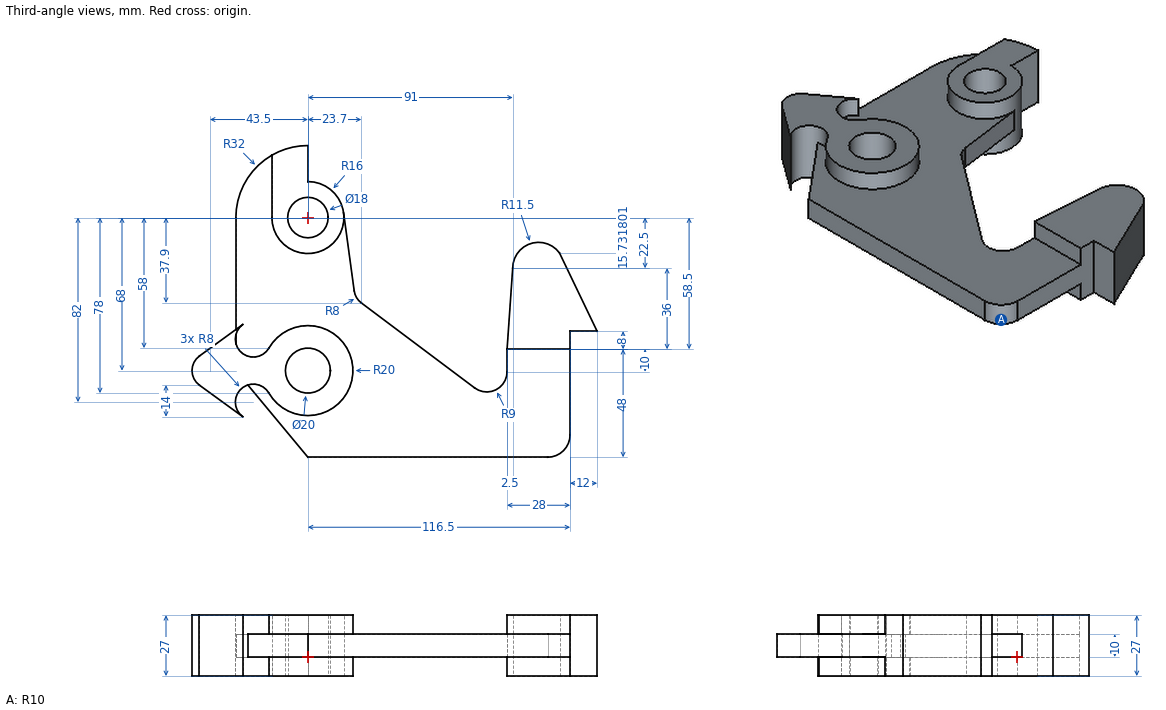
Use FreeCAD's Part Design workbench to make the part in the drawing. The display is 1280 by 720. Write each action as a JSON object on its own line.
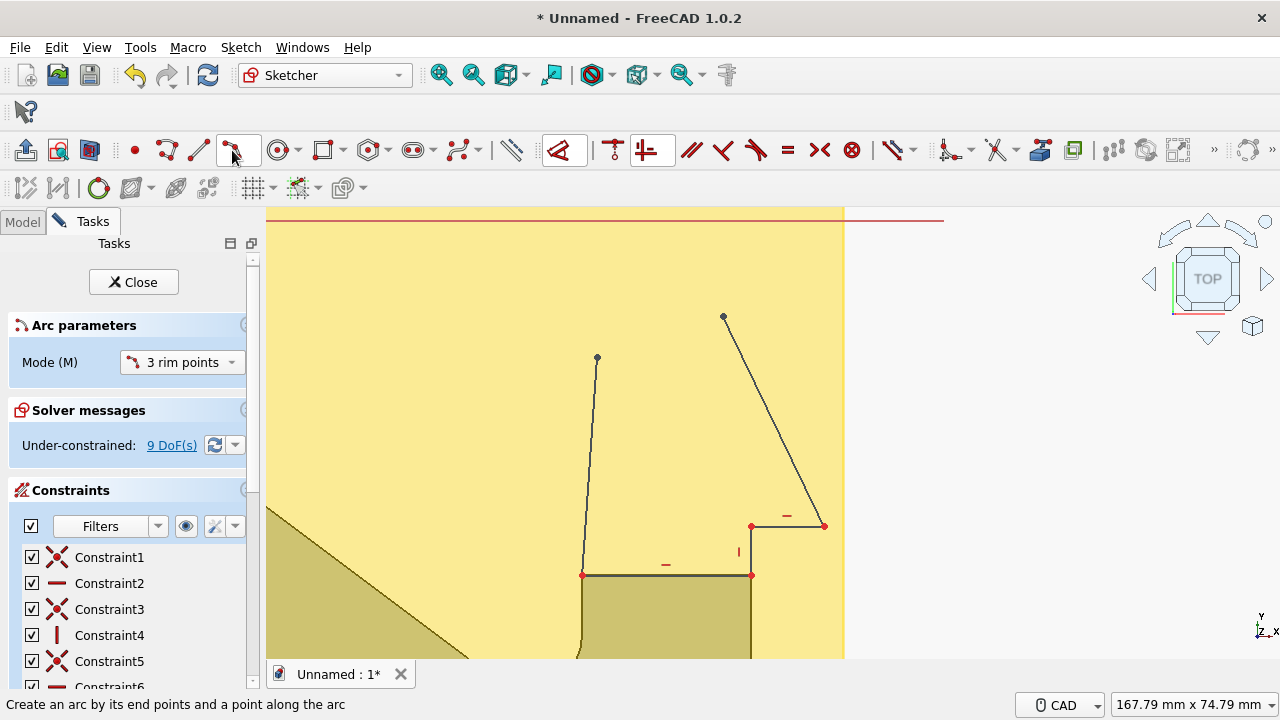
{"action": "left_click", "coordinate": [723, 317]}
{"action": "left_click", "coordinate": [597, 358]}
{"action": "left_click", "coordinate": [645, 291]}
{"action": "key", "text": "Escape"}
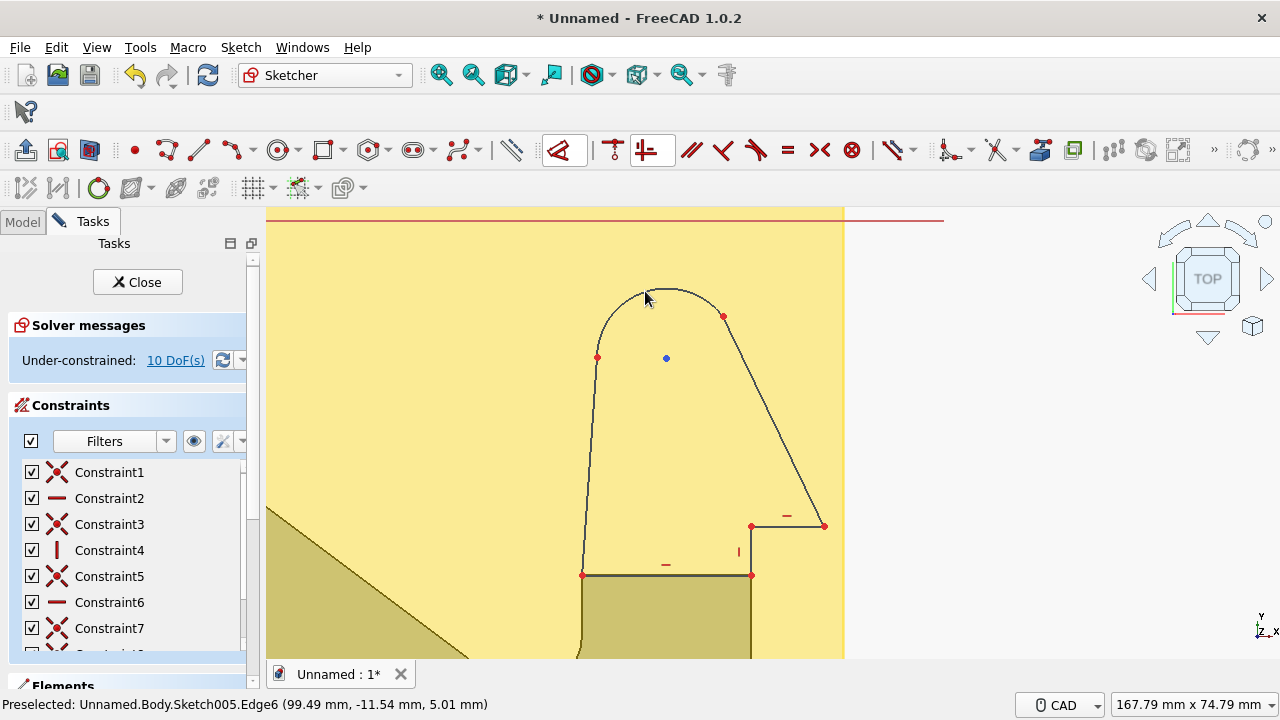
{"action": "left_click", "coordinate": [680, 290]}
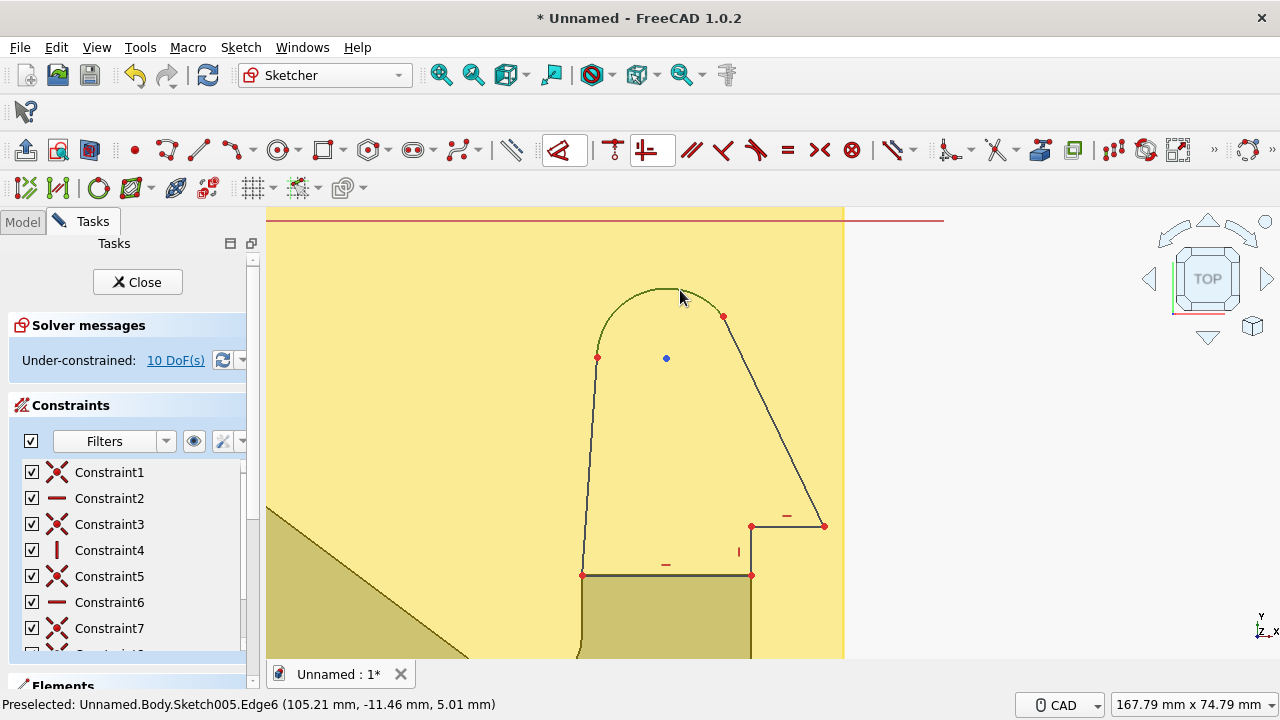
{"action": "key", "text": "k r"}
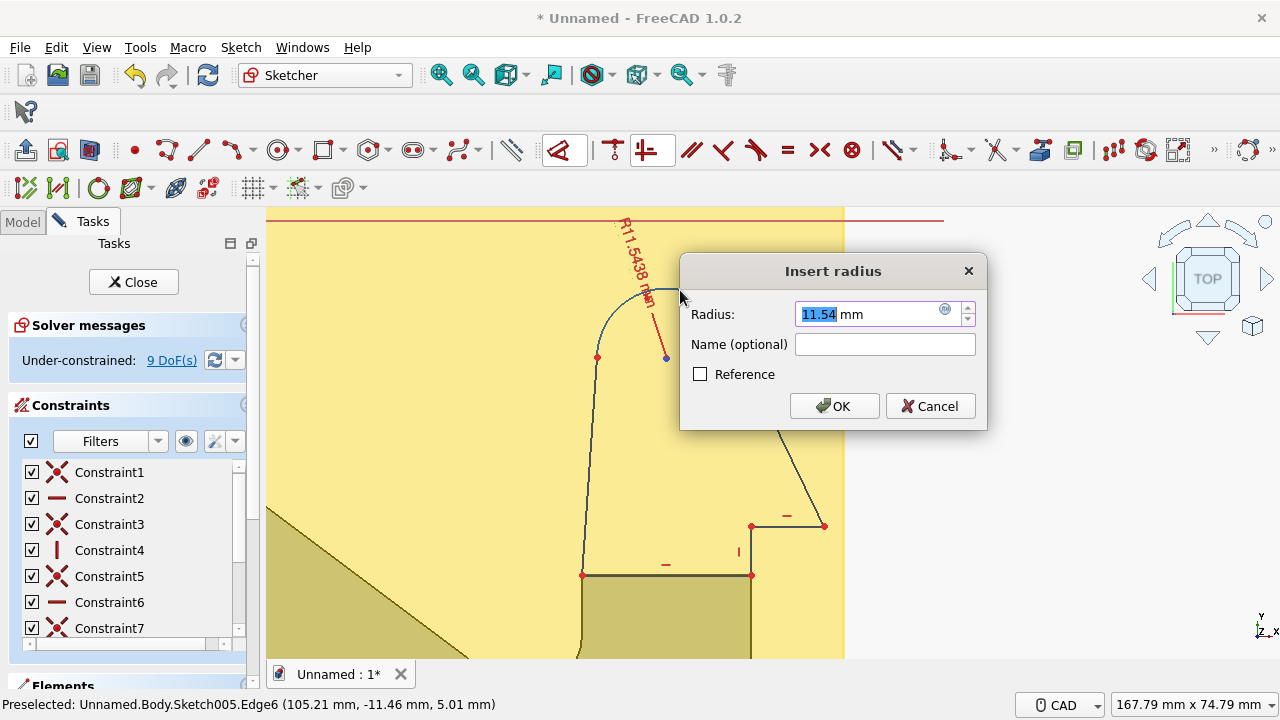
{"action": "type", "text": "11.5"}
{"action": "key", "text": "Return"}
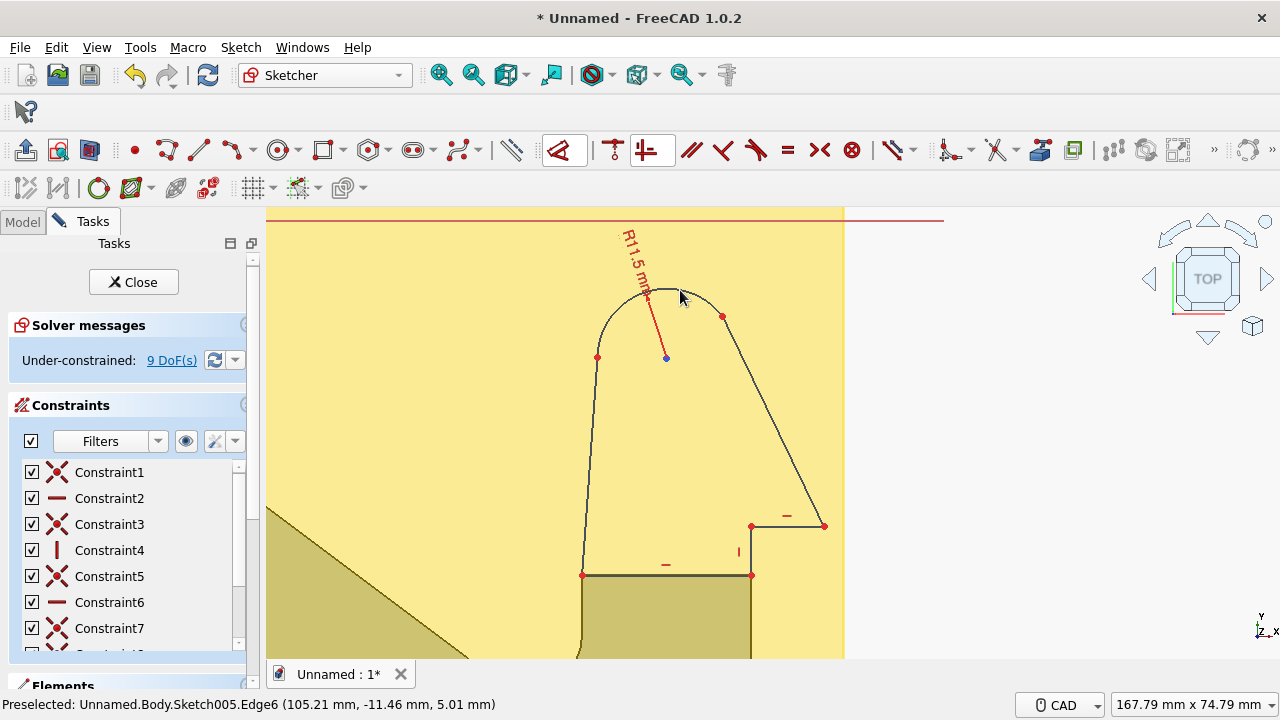
{"action": "left_click", "coordinate": [751, 561]}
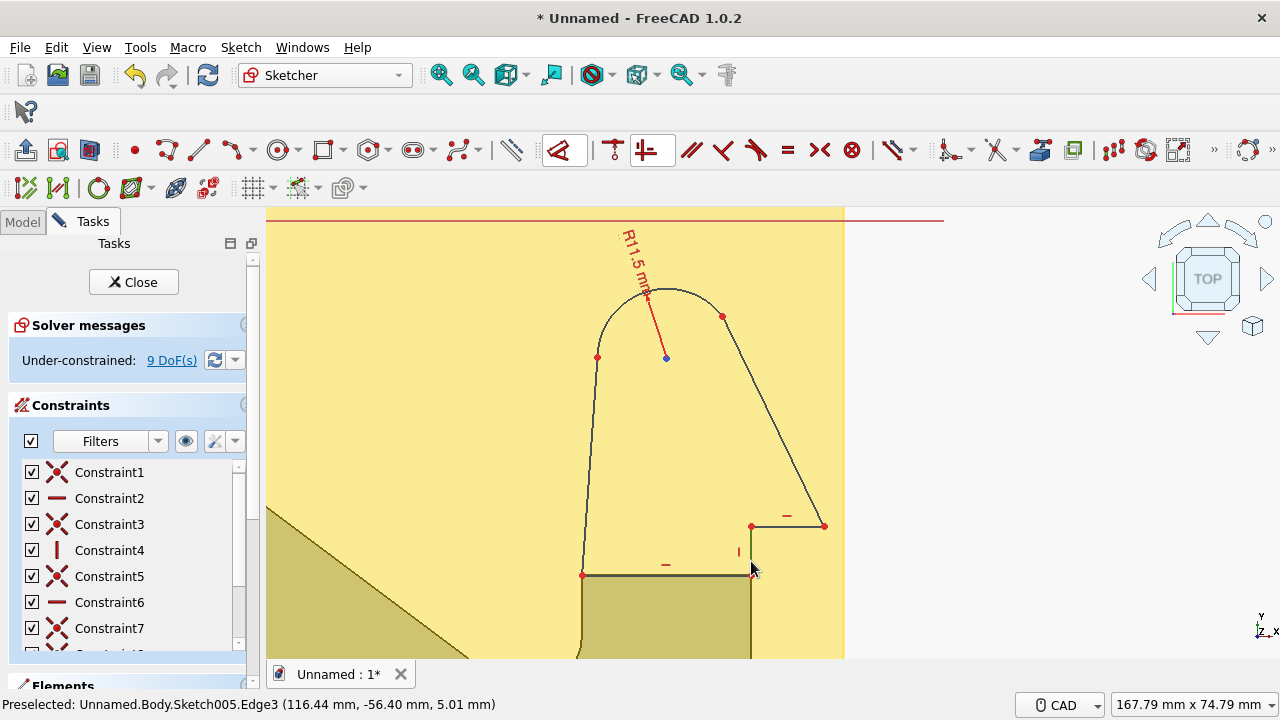
{"action": "key", "text": "i"}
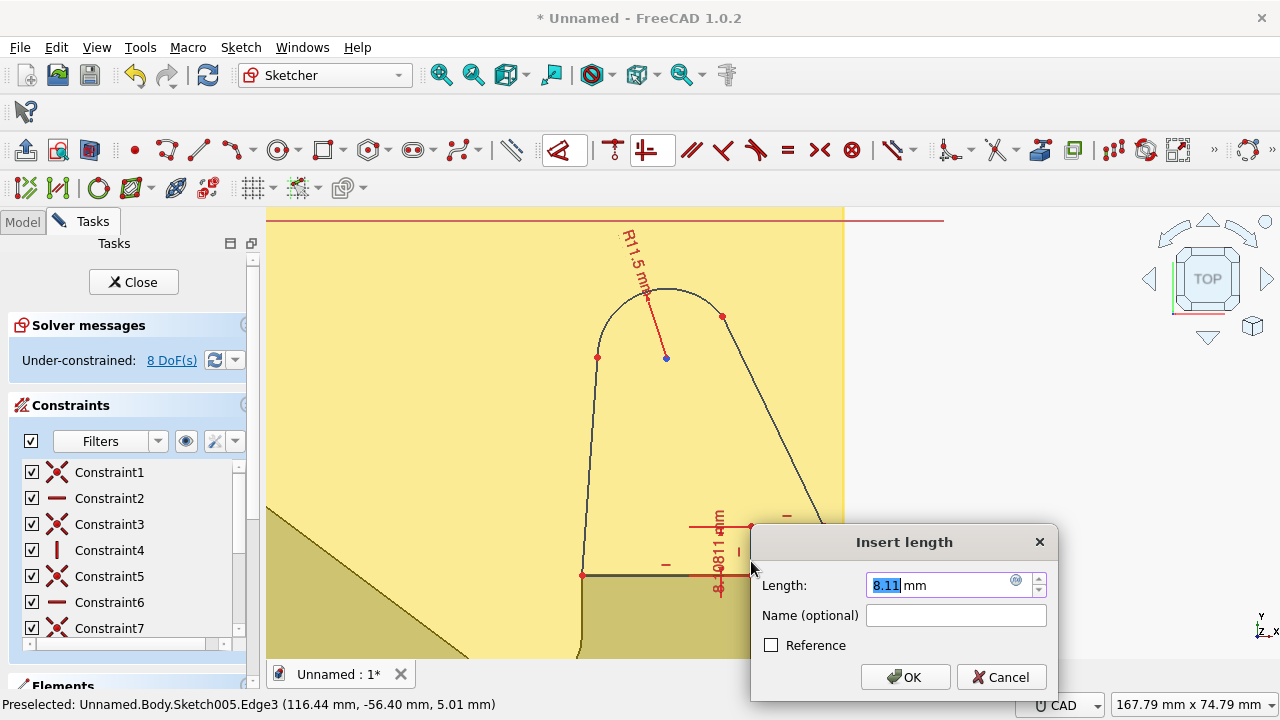
{"action": "type", "text": "8"}
{"action": "key", "text": "Return"}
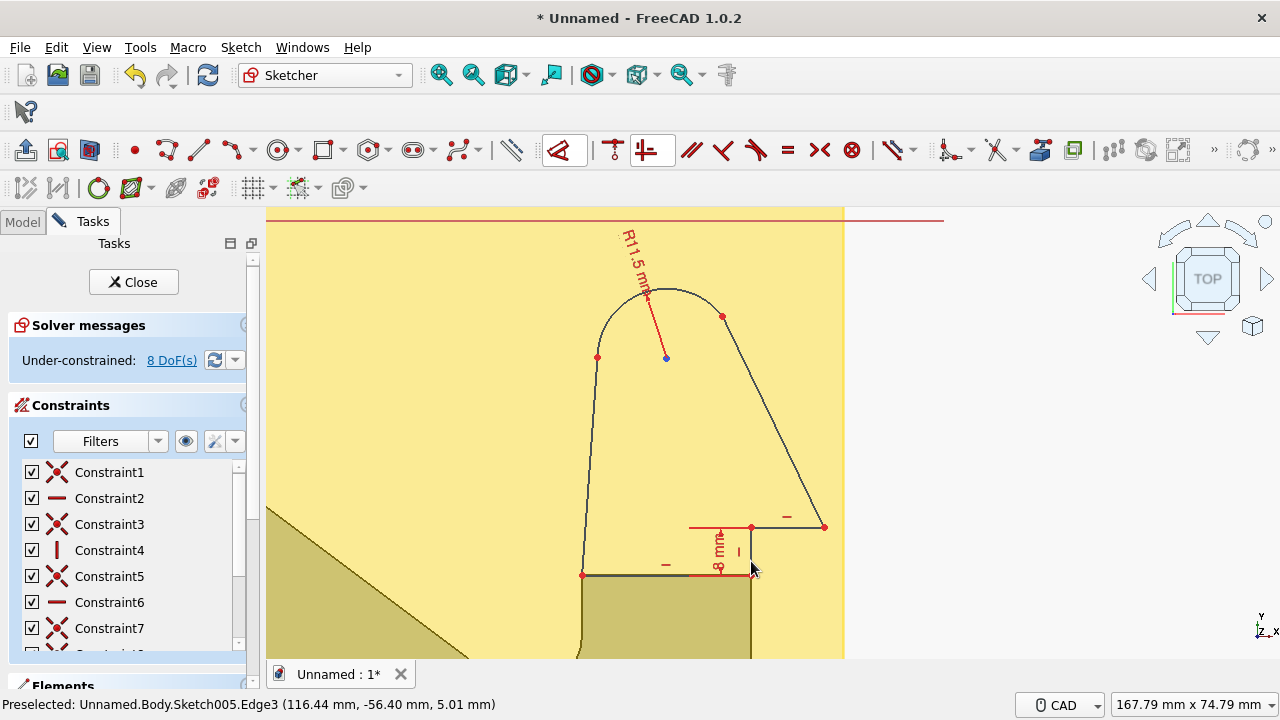
{"action": "left_click", "coordinate": [633, 576]}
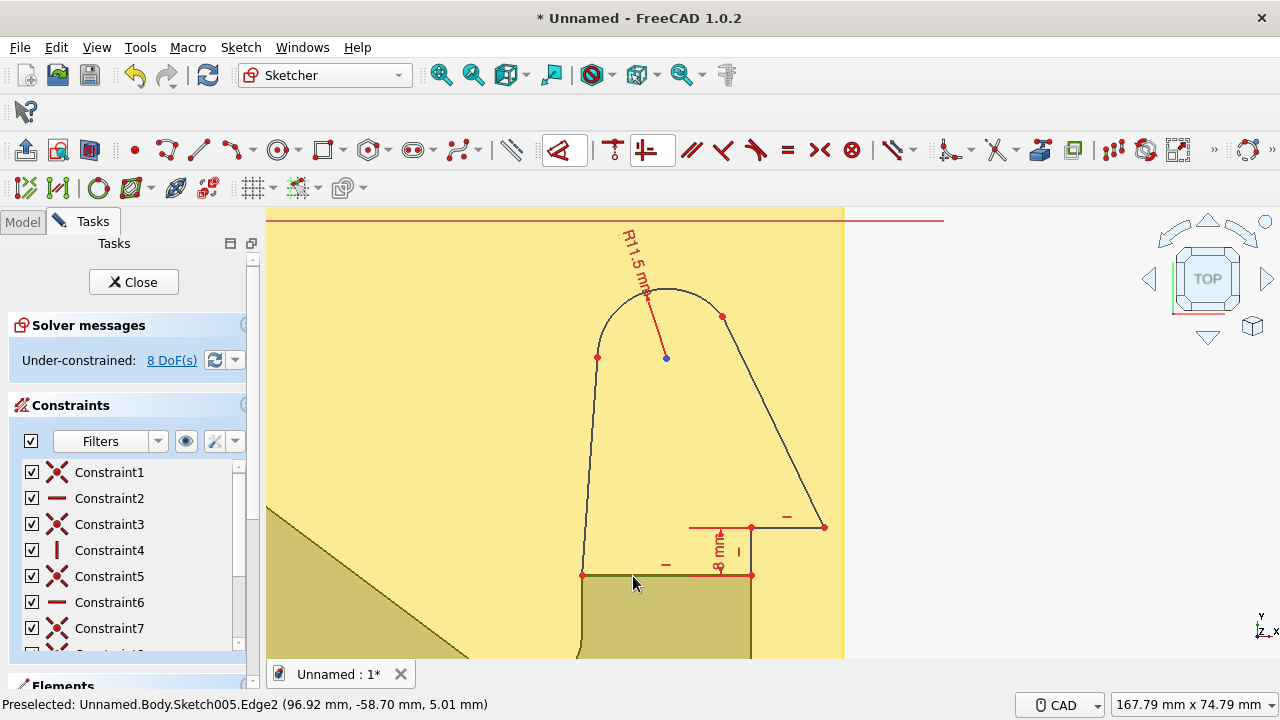
{"action": "left_click", "coordinate": [582, 150]}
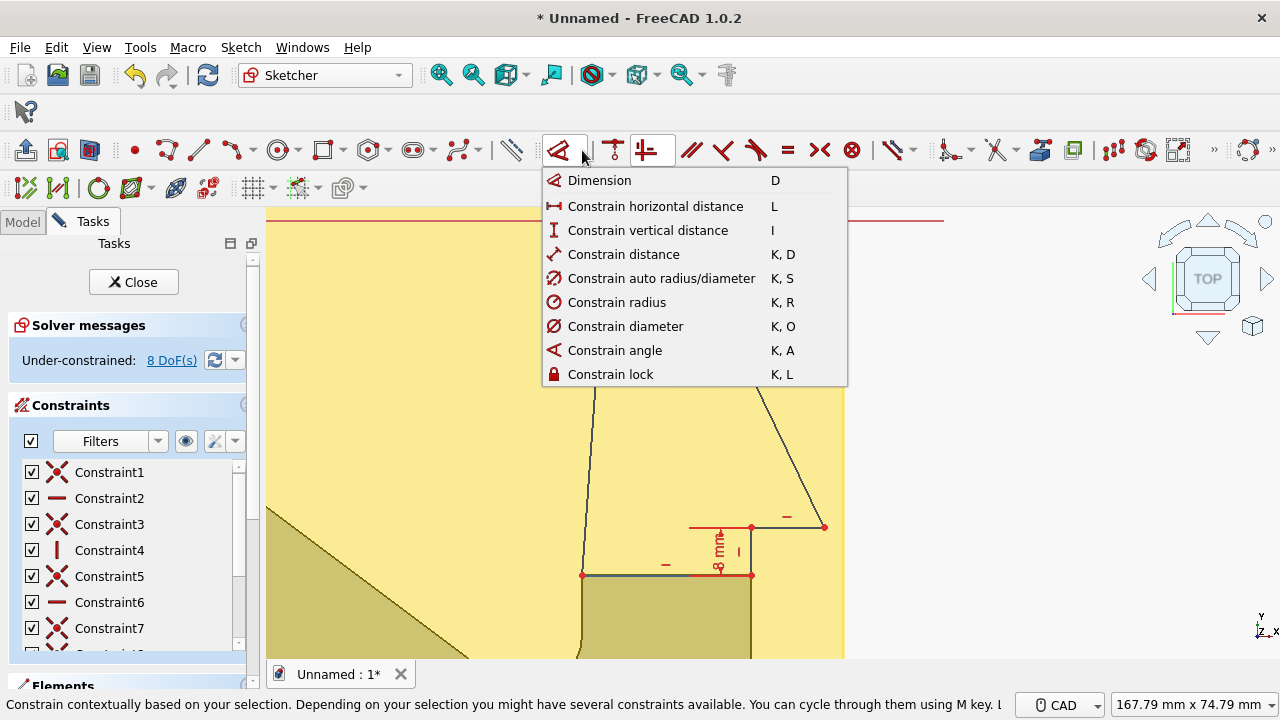
{"action": "left_click", "coordinate": [695, 206]}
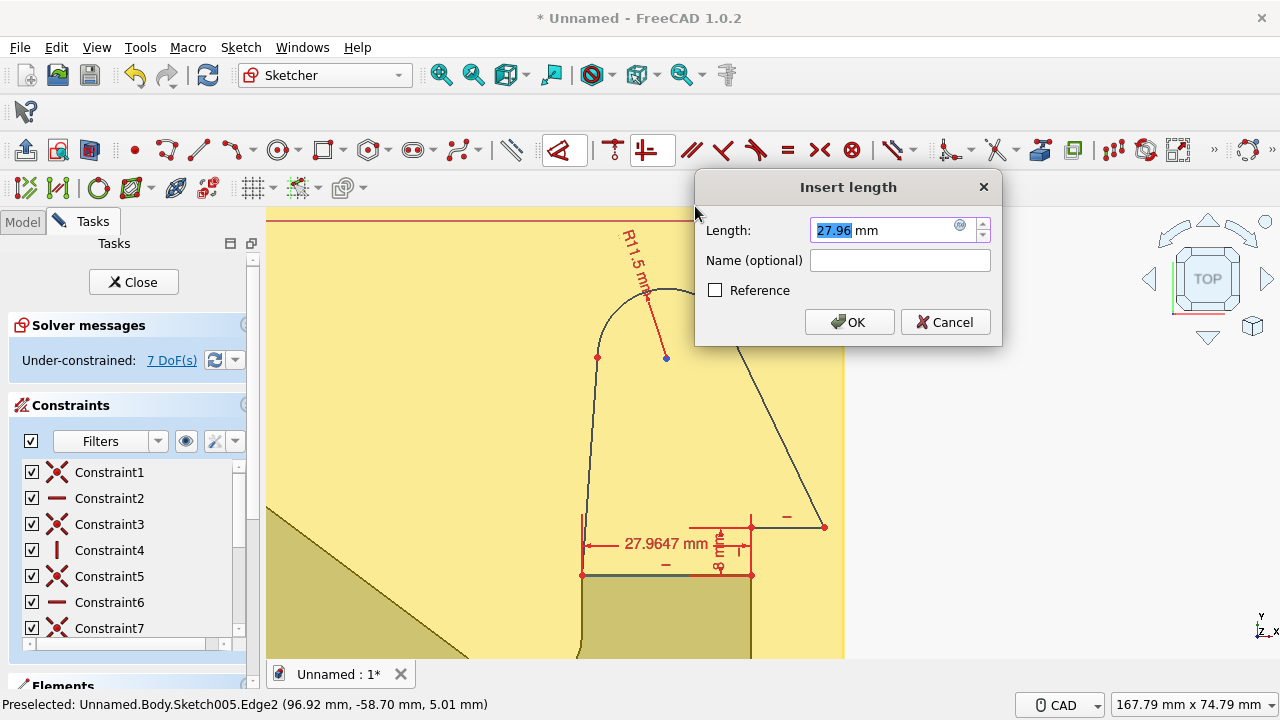
{"action": "type", "text": "28"}
{"action": "key", "text": "Return"}